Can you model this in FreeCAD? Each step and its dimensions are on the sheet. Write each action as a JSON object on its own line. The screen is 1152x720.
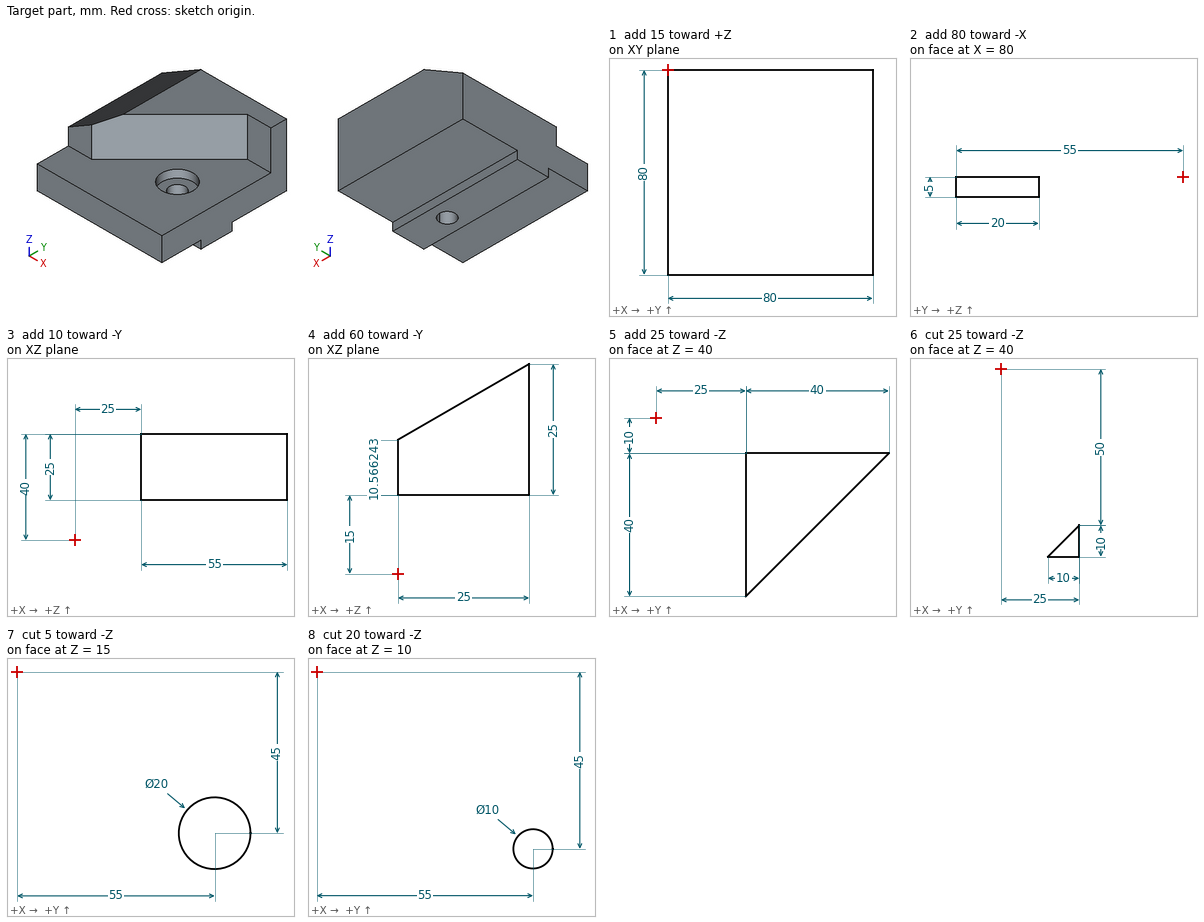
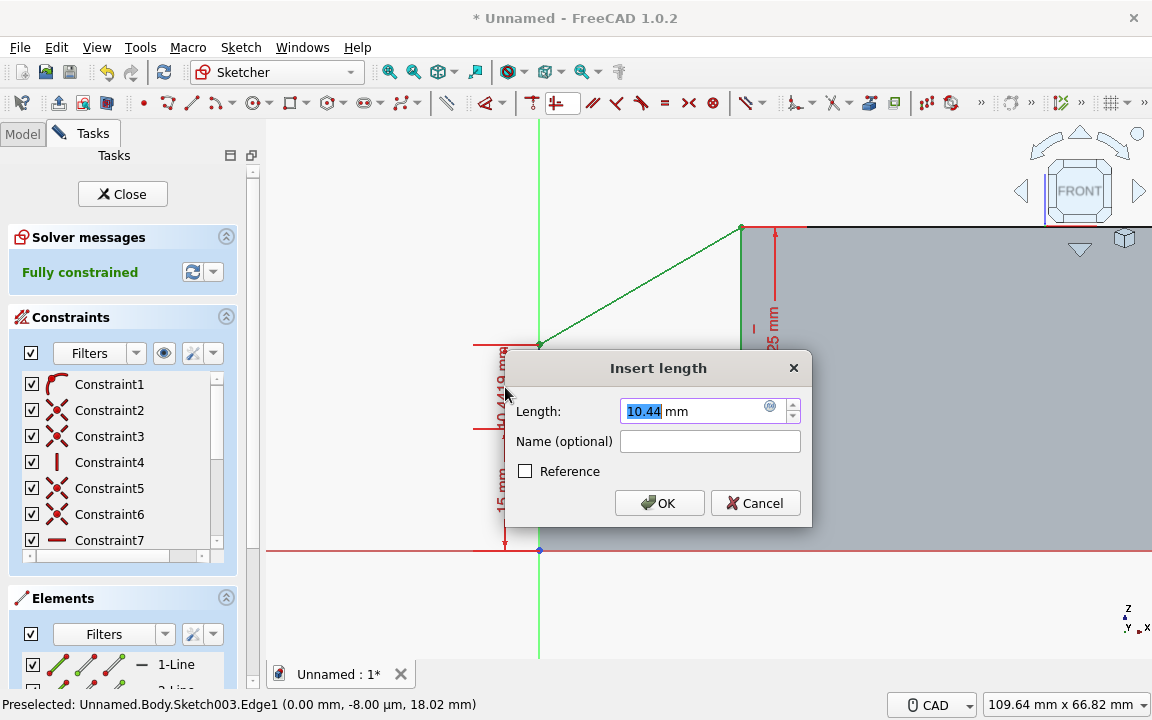
{"action": "type", "text": "10.566243"}
{"action": "key", "text": "Return"}
{"action": "key", "text": "Escape"}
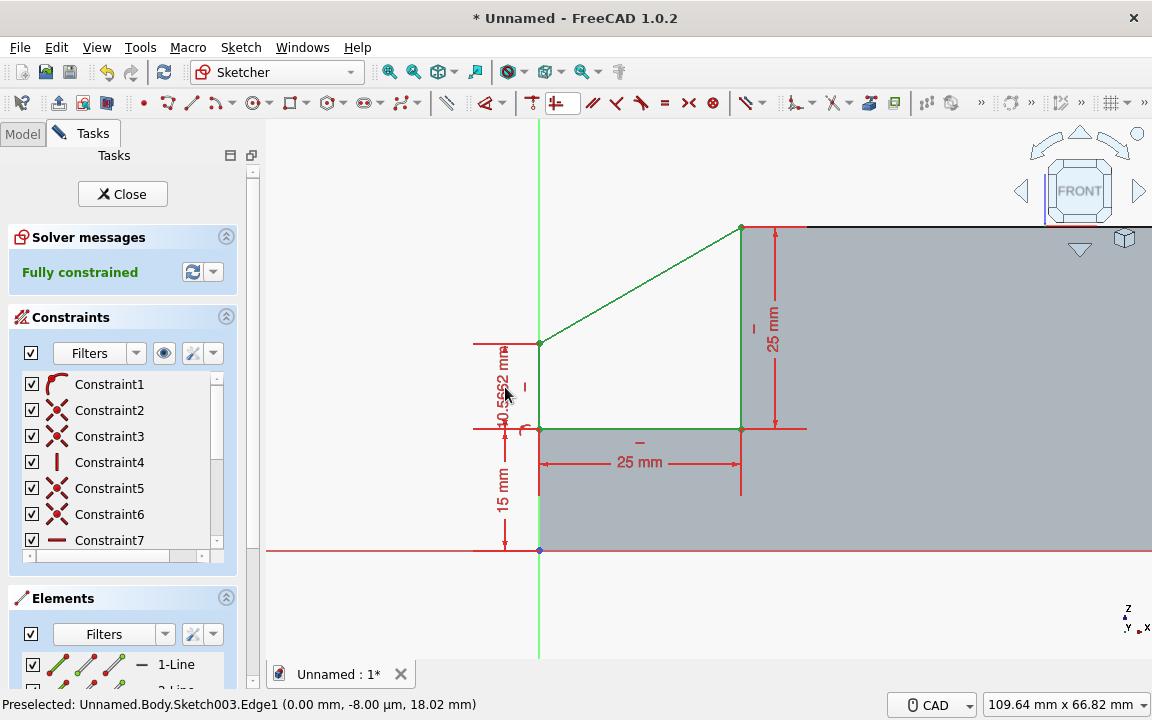
{"action": "left_click", "coordinate": [123, 194]}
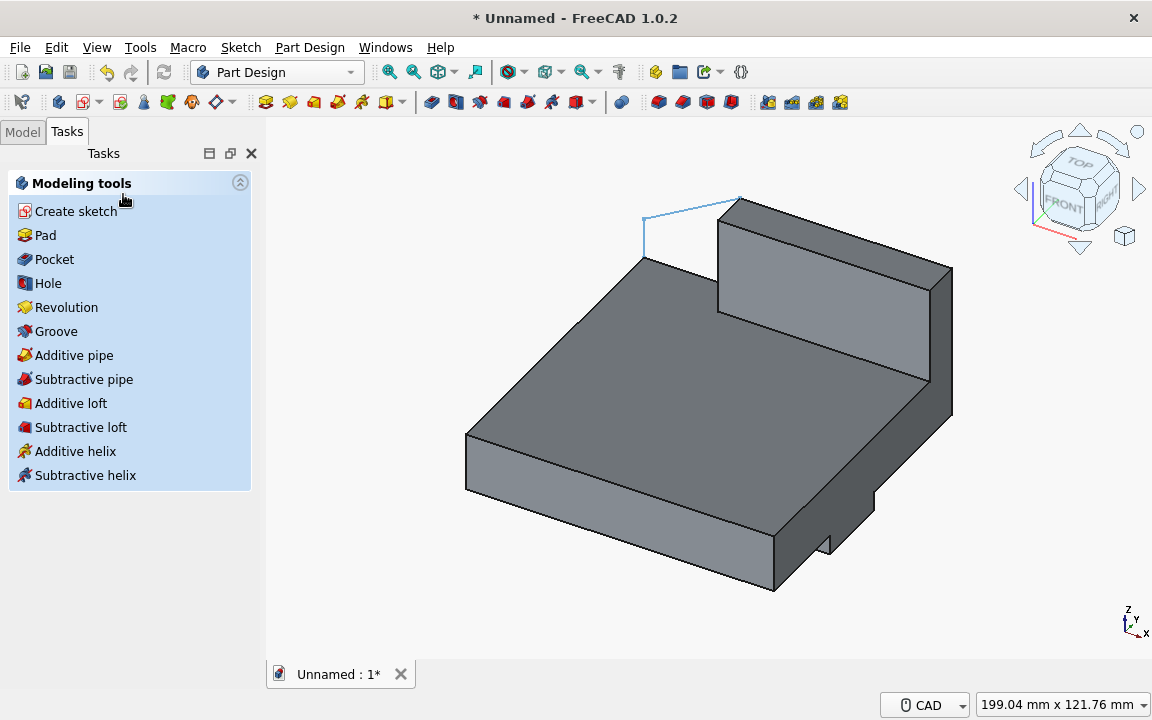
{"action": "left_click", "coordinate": [266, 102]}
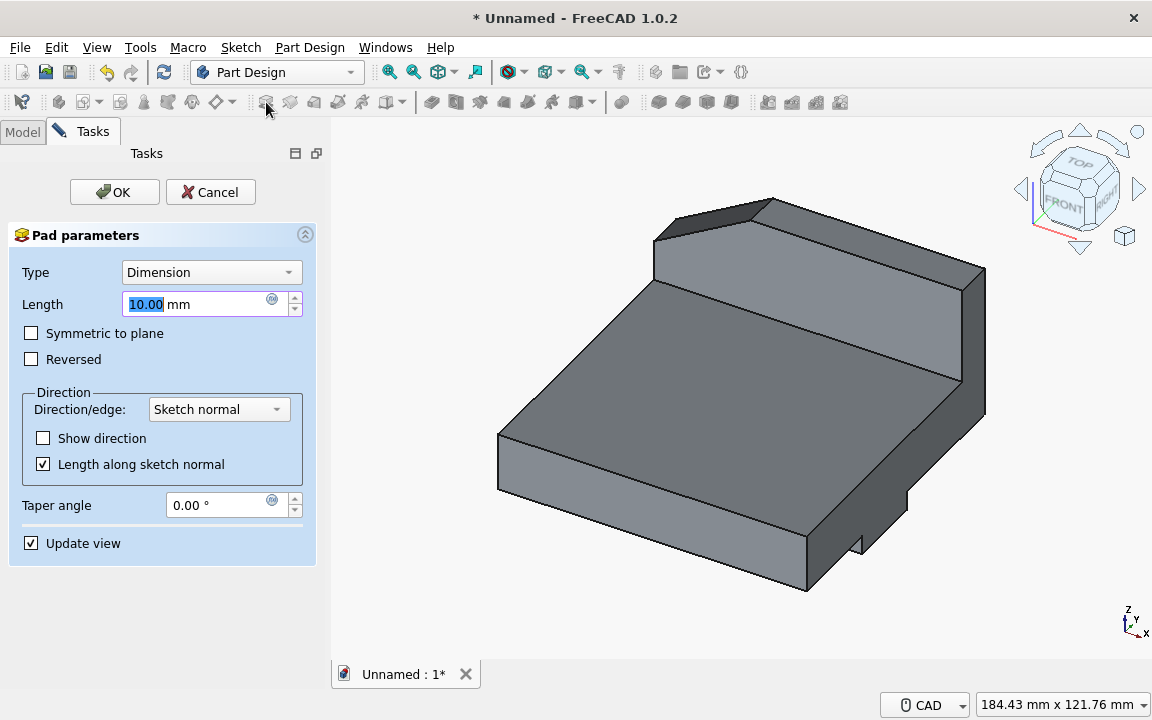
{"action": "type", "text": "60"}
{"action": "key", "text": "Tab"}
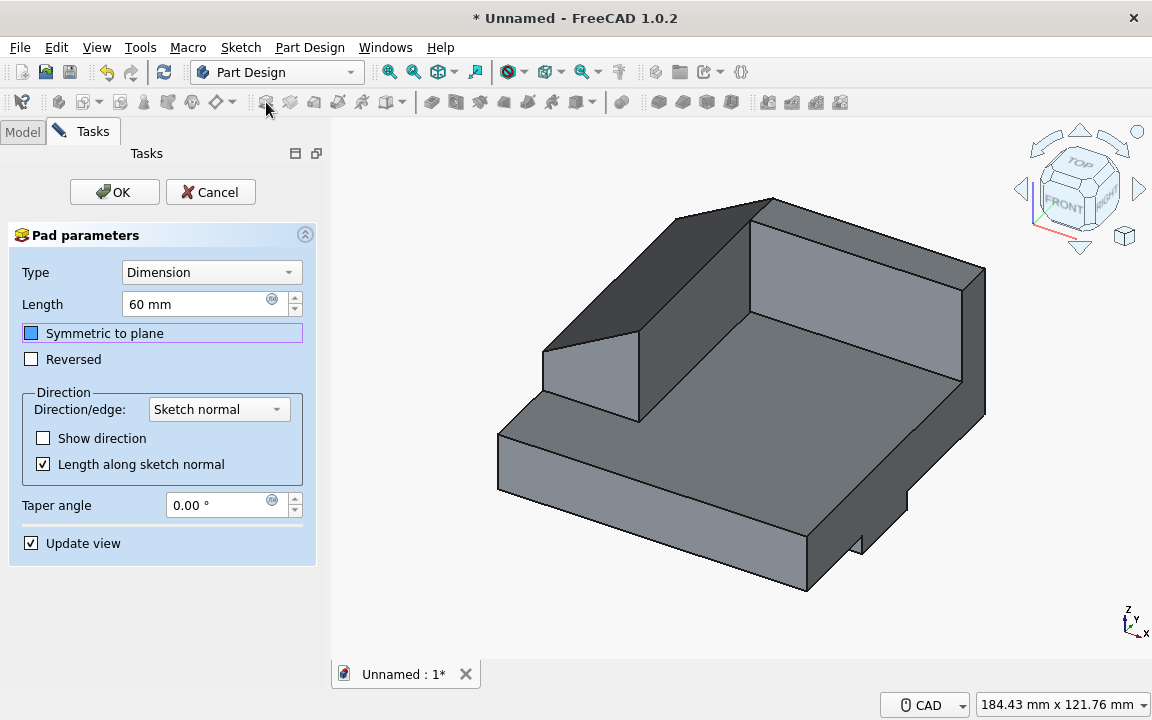
{"action": "left_click", "coordinate": [115, 192]}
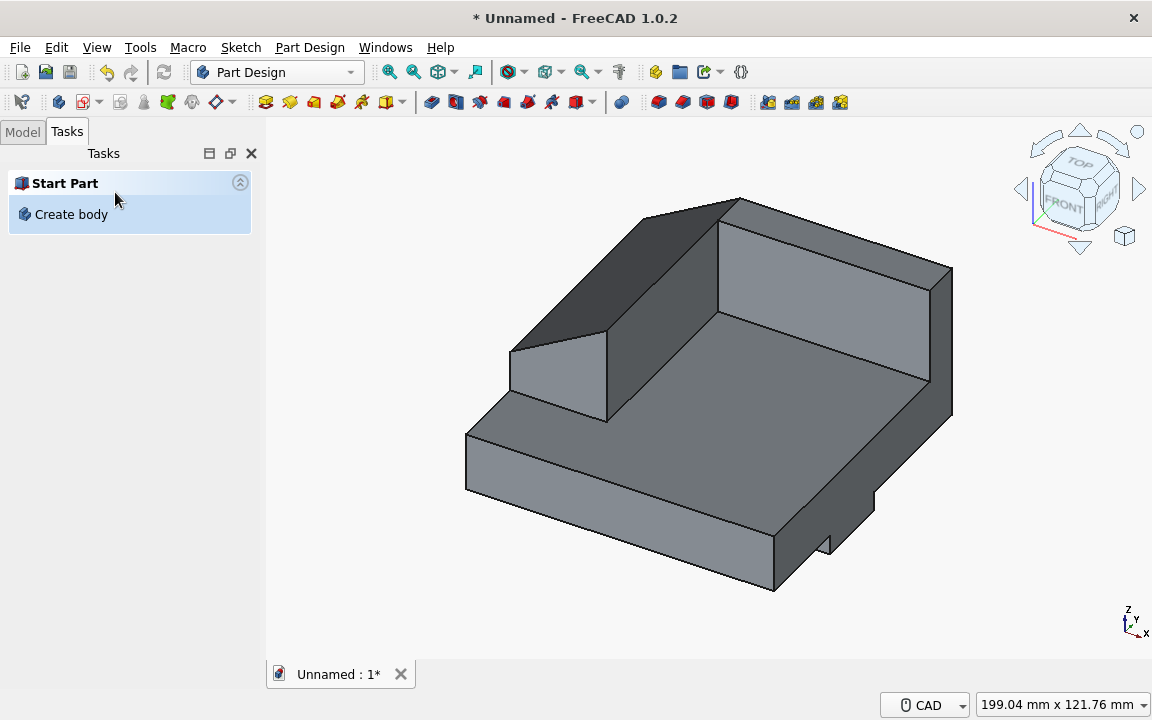
{"action": "left_click", "coordinate": [896, 264]}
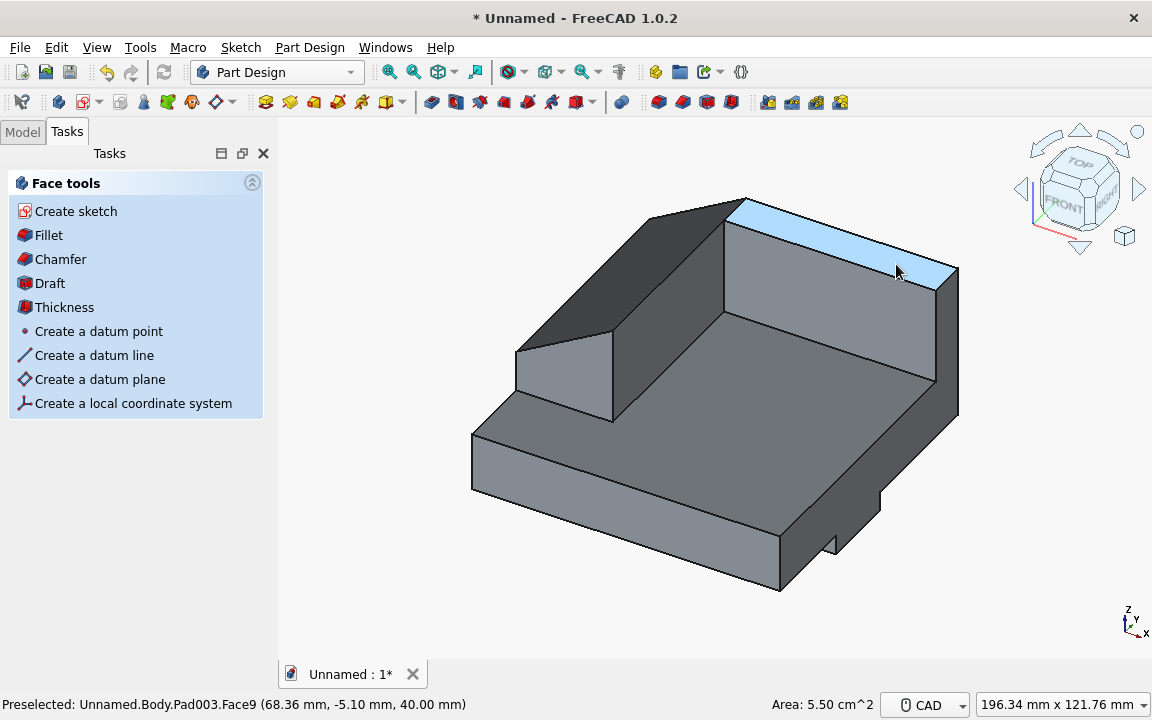
{"action": "left_click", "coordinate": [84, 102]}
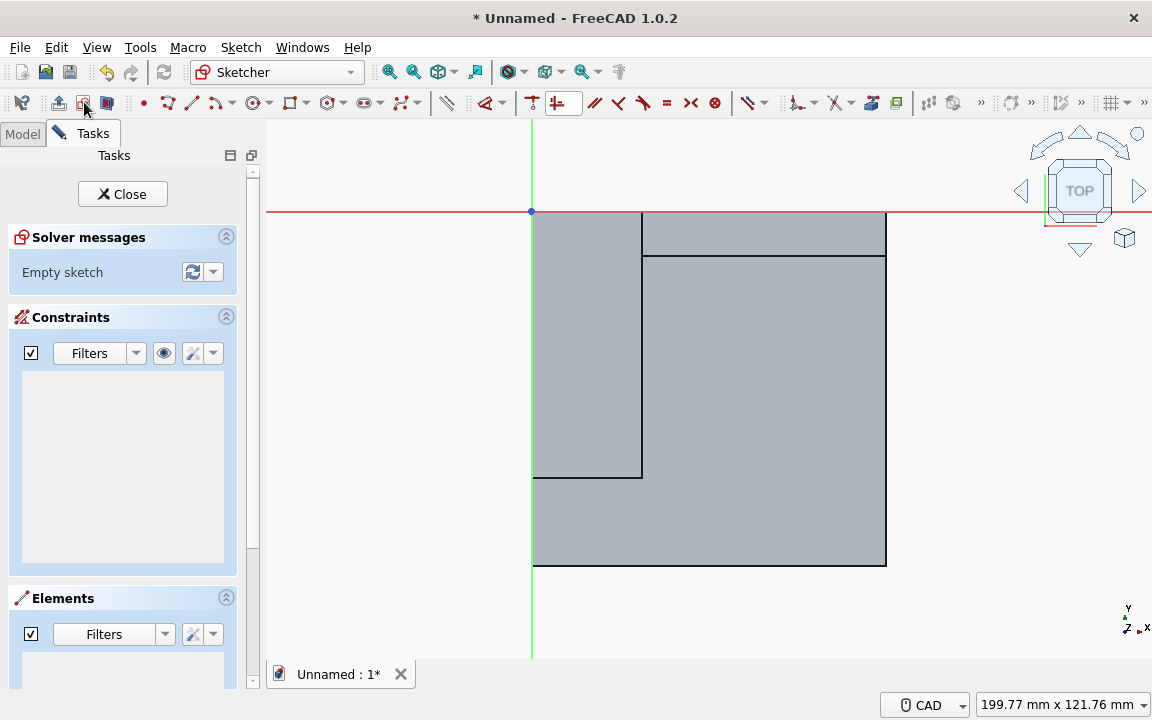
{"action": "scroll", "coordinate": [747, 187], "scroll_direction": "up", "scroll_amount": 2}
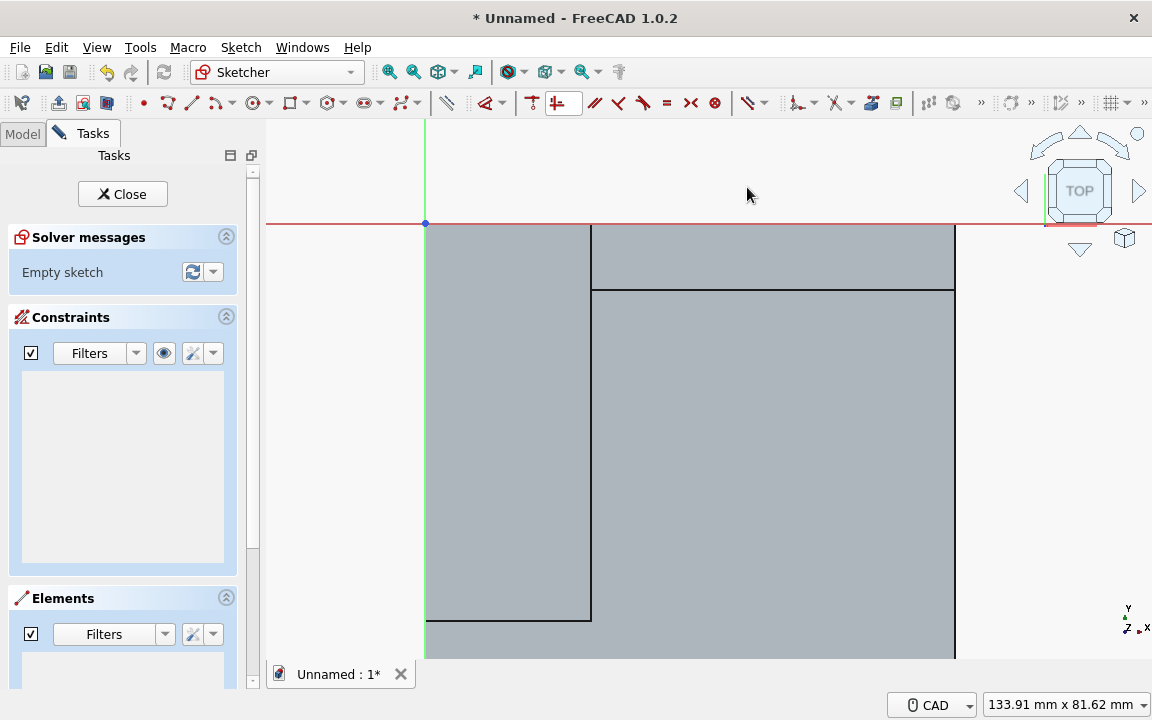
{"action": "left_click", "coordinate": [168, 104]}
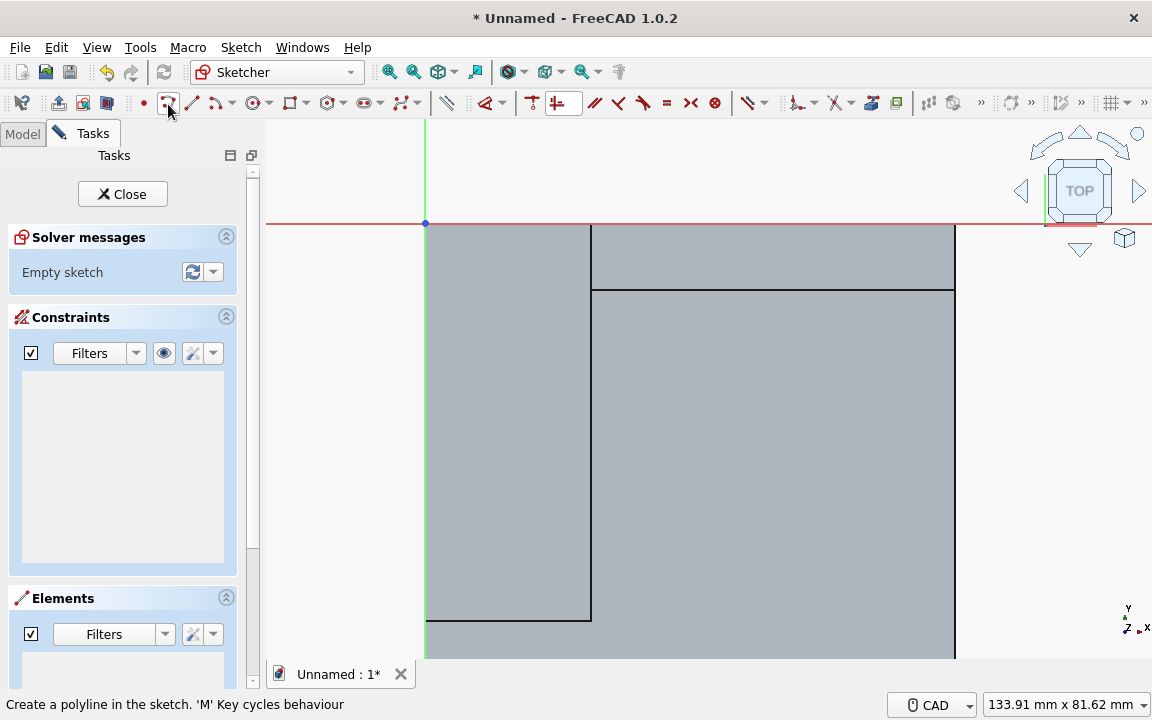
{"action": "left_click", "coordinate": [591, 290]}
{"action": "left_click", "coordinate": [591, 554]}
{"action": "left_click", "coordinate": [855, 290]}
{"action": "left_click", "coordinate": [591, 291]}
{"action": "key", "text": "Escape"}
{"action": "key", "text": "Escape"}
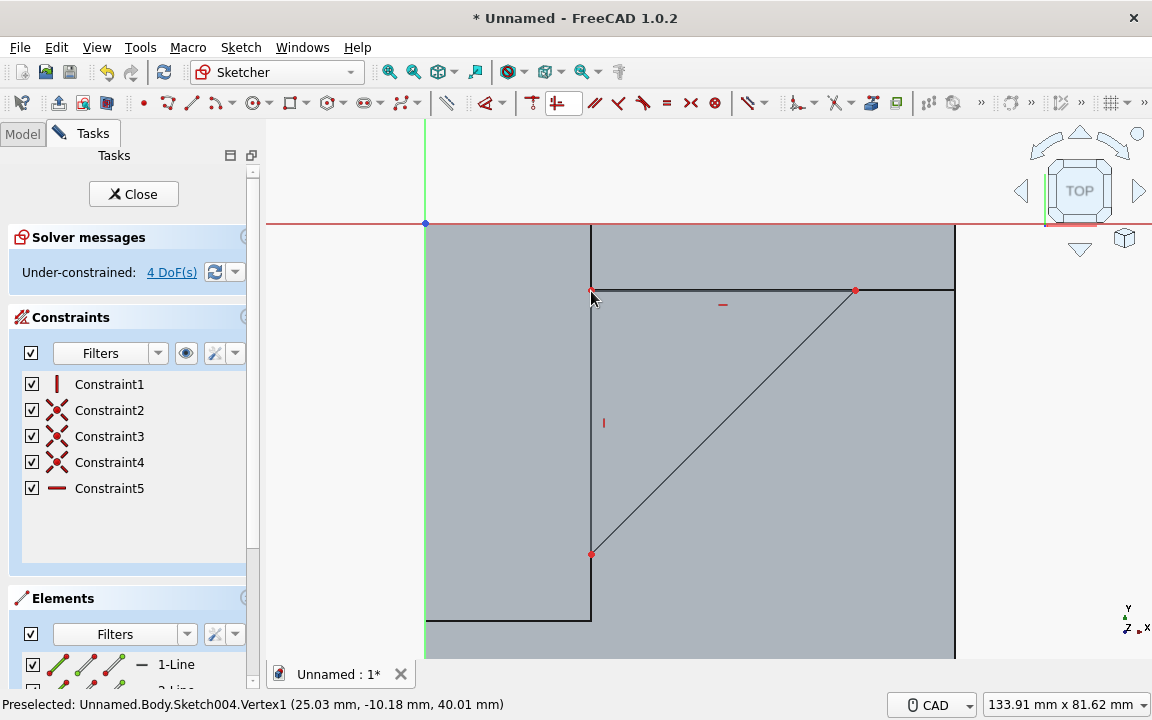
{"action": "left_click", "coordinate": [486, 104]}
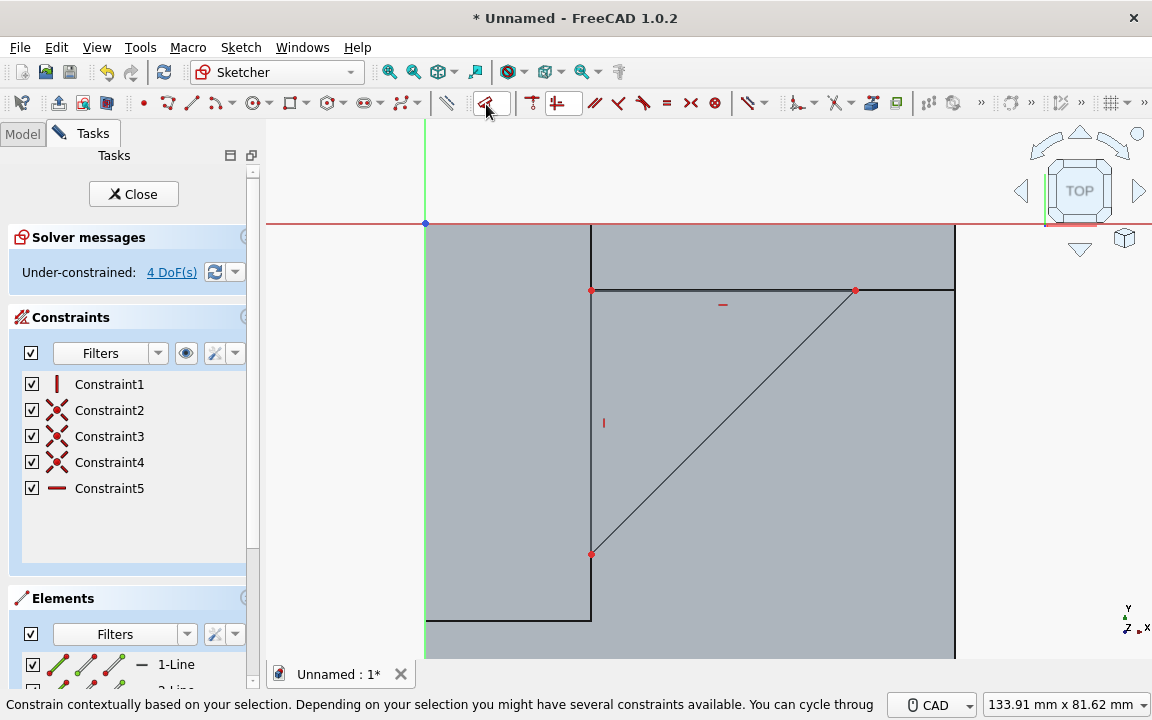
{"action": "left_click", "coordinate": [591, 370]}
{"action": "left_click", "coordinate": [557, 423]}